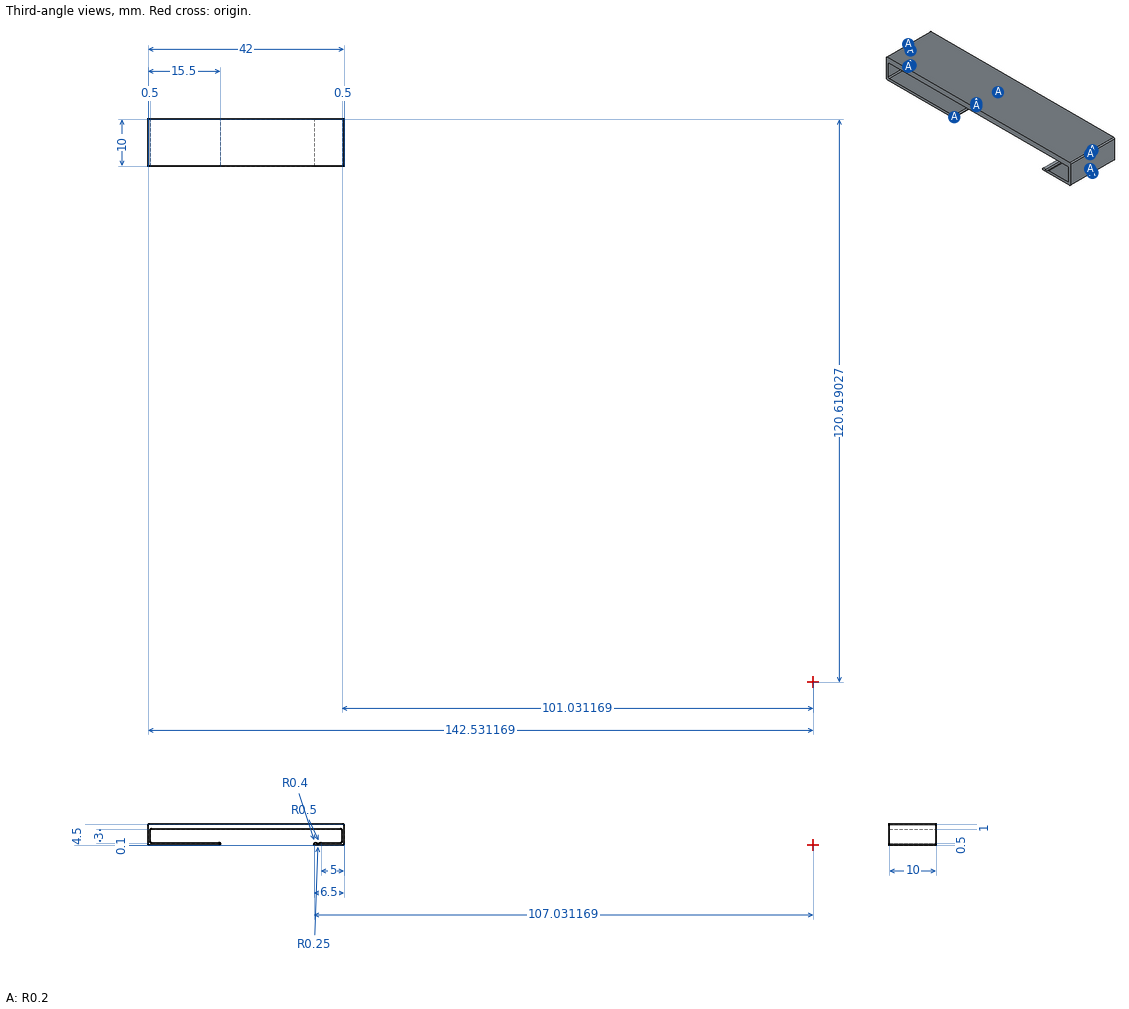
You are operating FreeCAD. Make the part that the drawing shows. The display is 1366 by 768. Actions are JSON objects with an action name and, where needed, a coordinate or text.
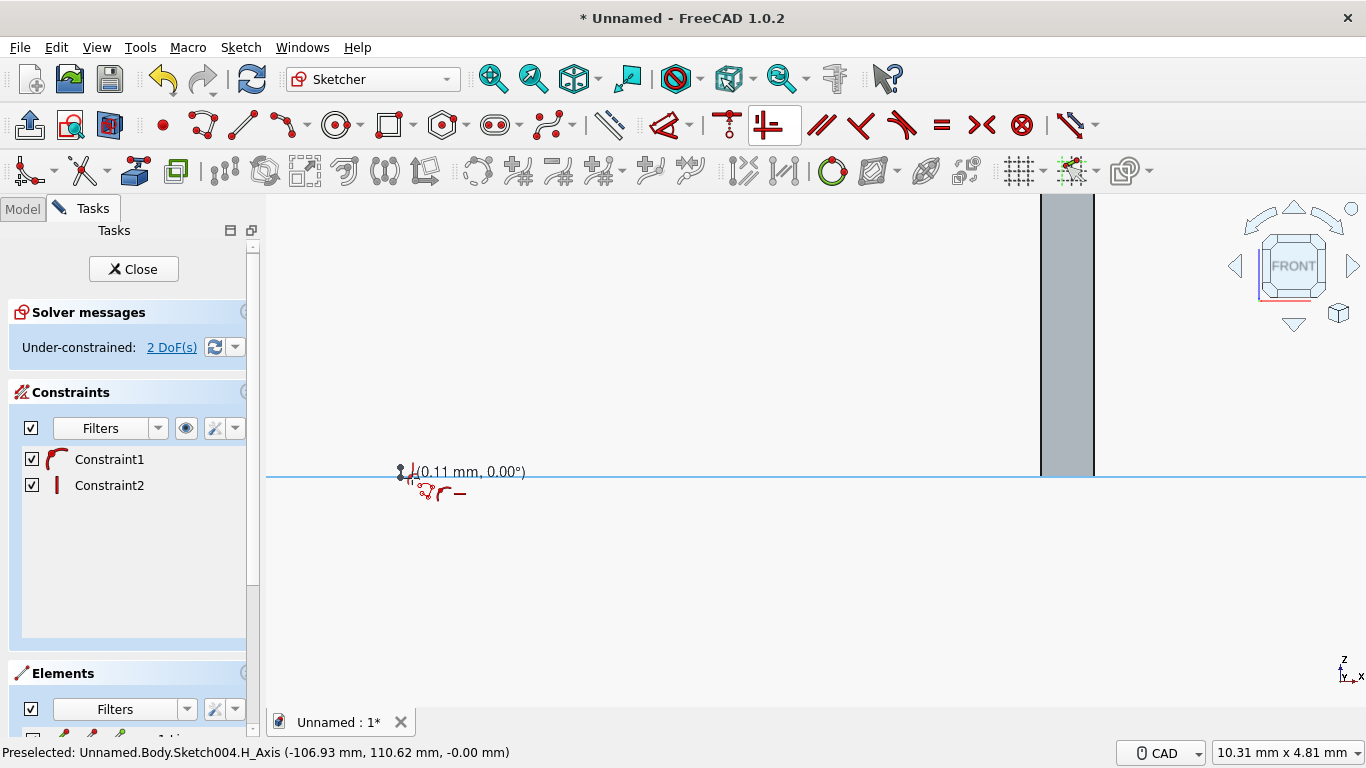
{"action": "left_click", "coordinate": [1094, 468]}
{"action": "left_click", "coordinate": [1094, 424]}
{"action": "left_click", "coordinate": [561, 424]}
{"action": "right_click", "coordinate": [561, 424]}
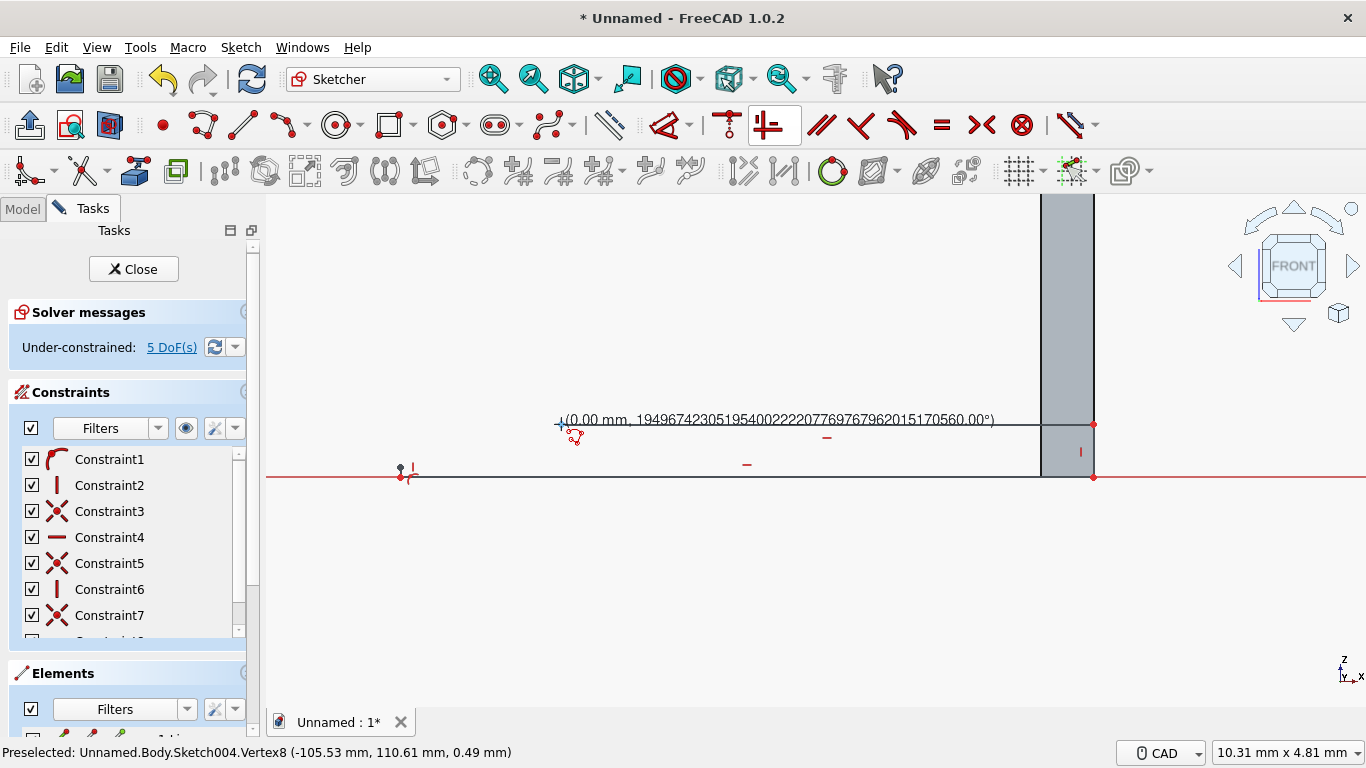
{"action": "left_click", "coordinate": [284, 126]}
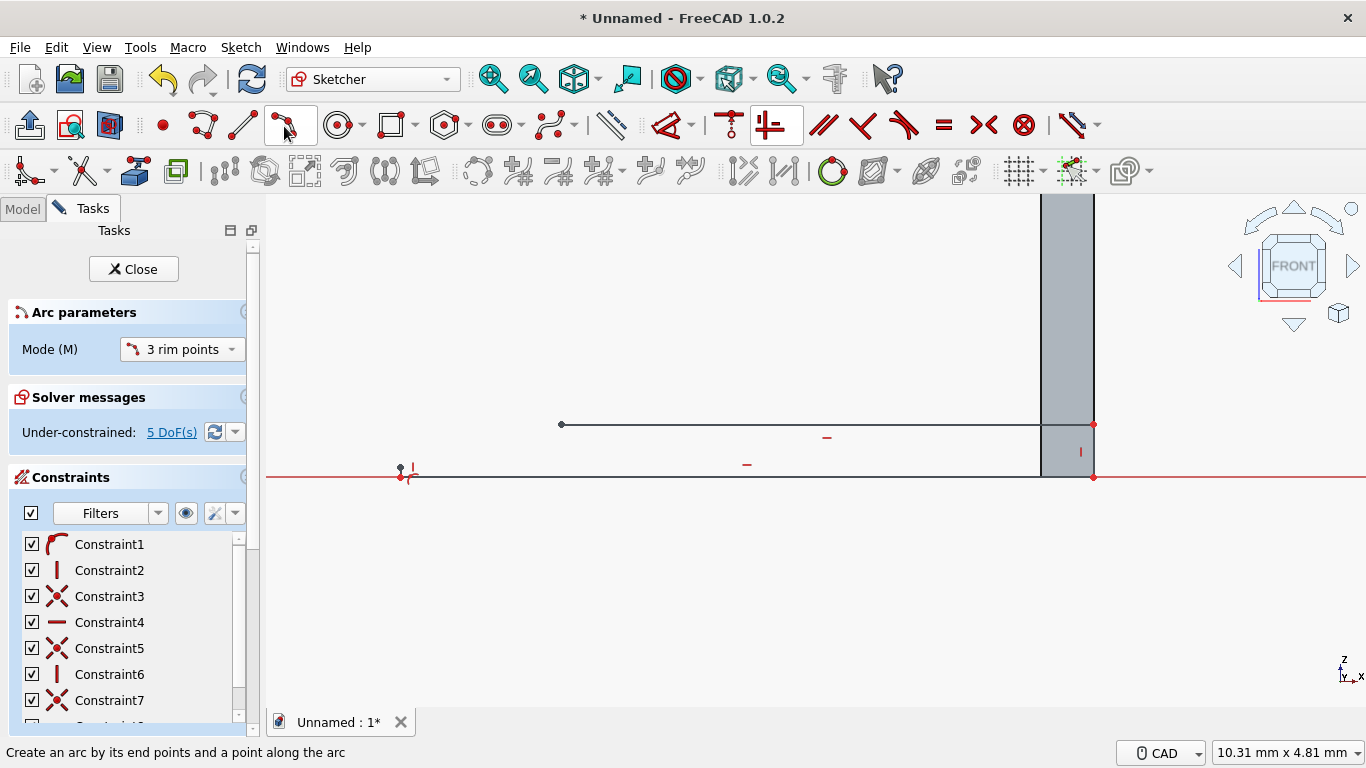
{"action": "left_click", "coordinate": [561, 425]}
{"action": "left_click", "coordinate": [520, 443]}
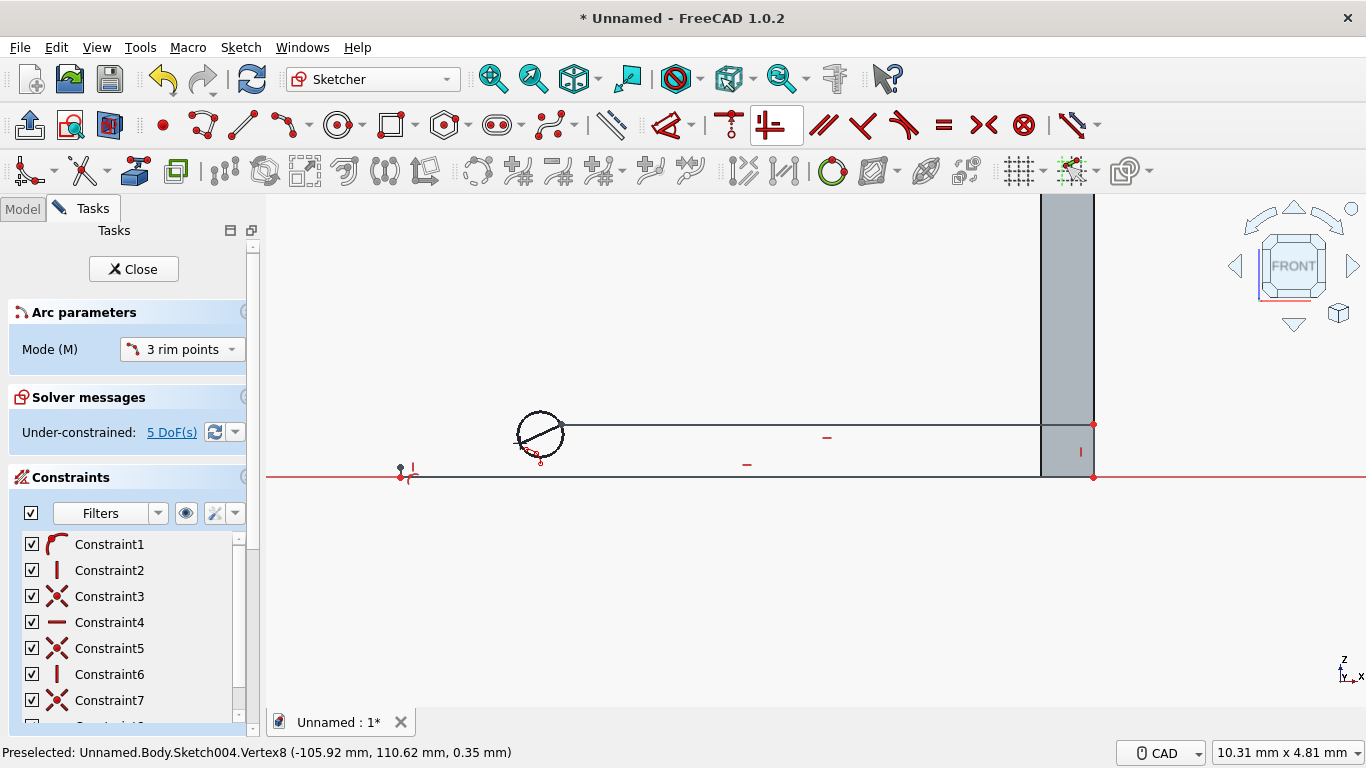
{"action": "scroll", "coordinate": [538, 429], "scroll_direction": "up", "scroll_amount": 6}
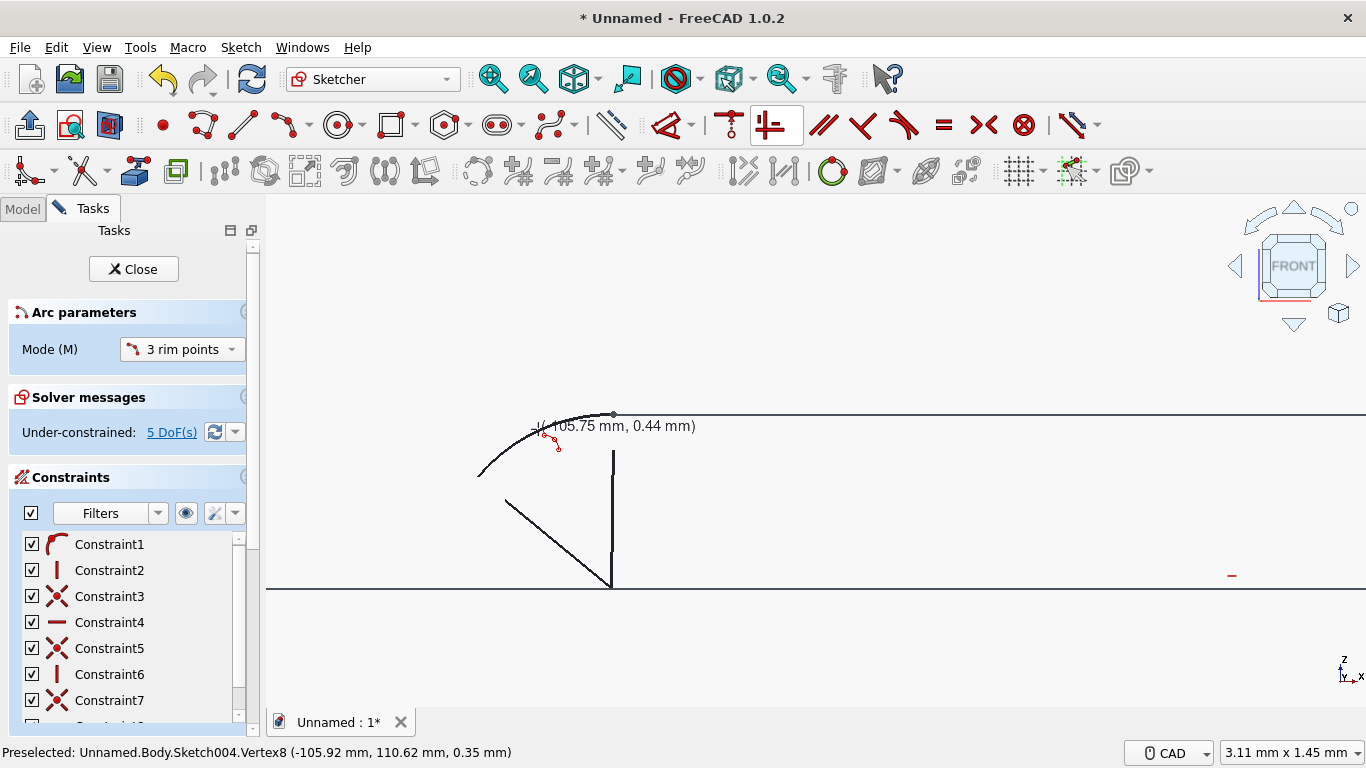
{"action": "left_click", "coordinate": [538, 428]}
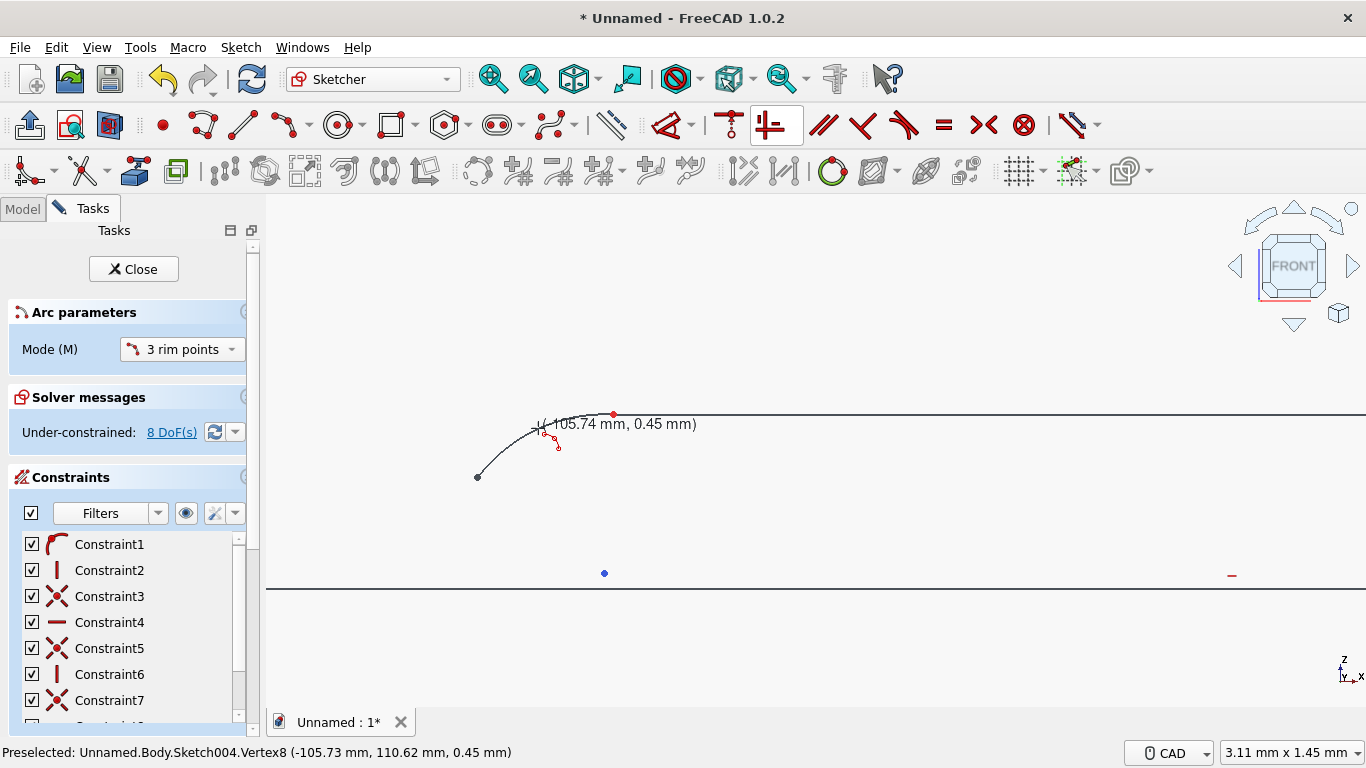
{"action": "left_click", "coordinate": [478, 478]}
{"action": "left_click", "coordinate": [338, 470]}
{"action": "left_click", "coordinate": [407, 506]}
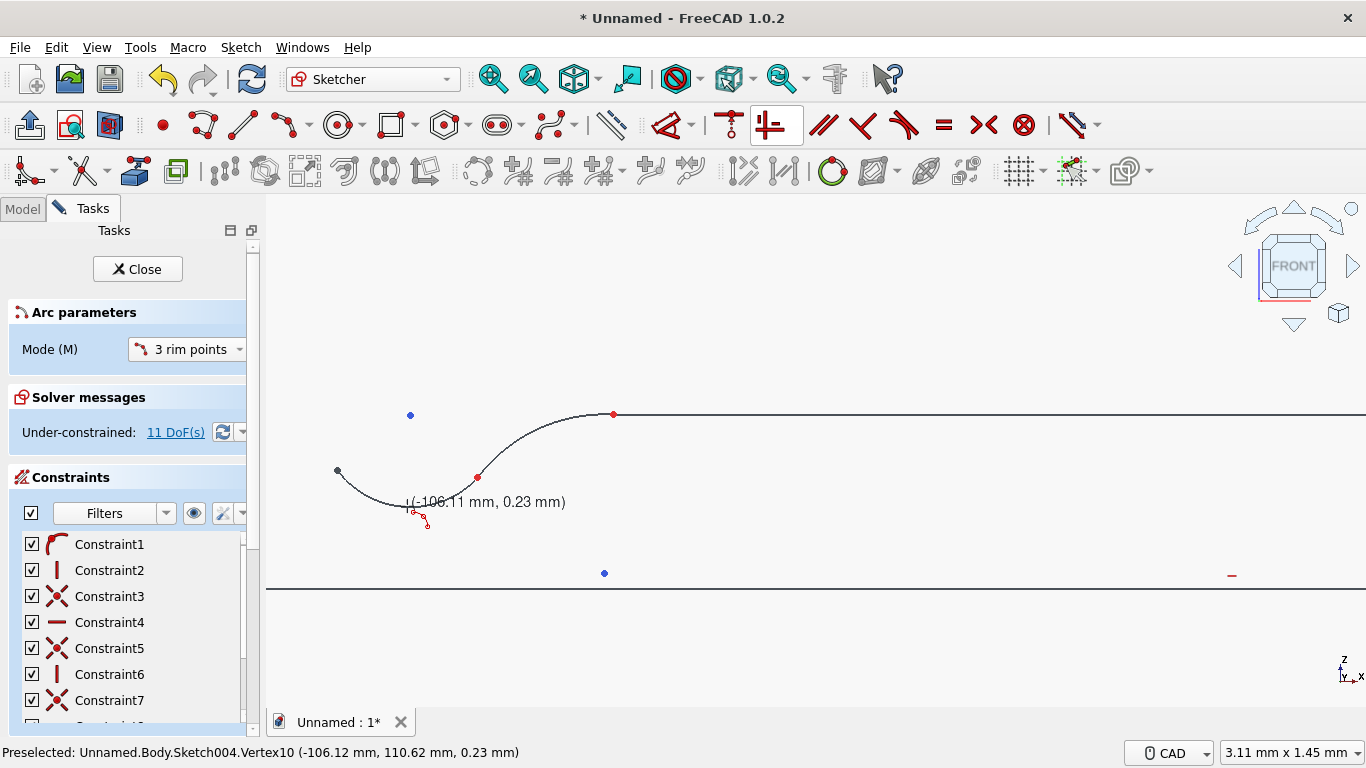
{"action": "left_click", "coordinate": [338, 471]}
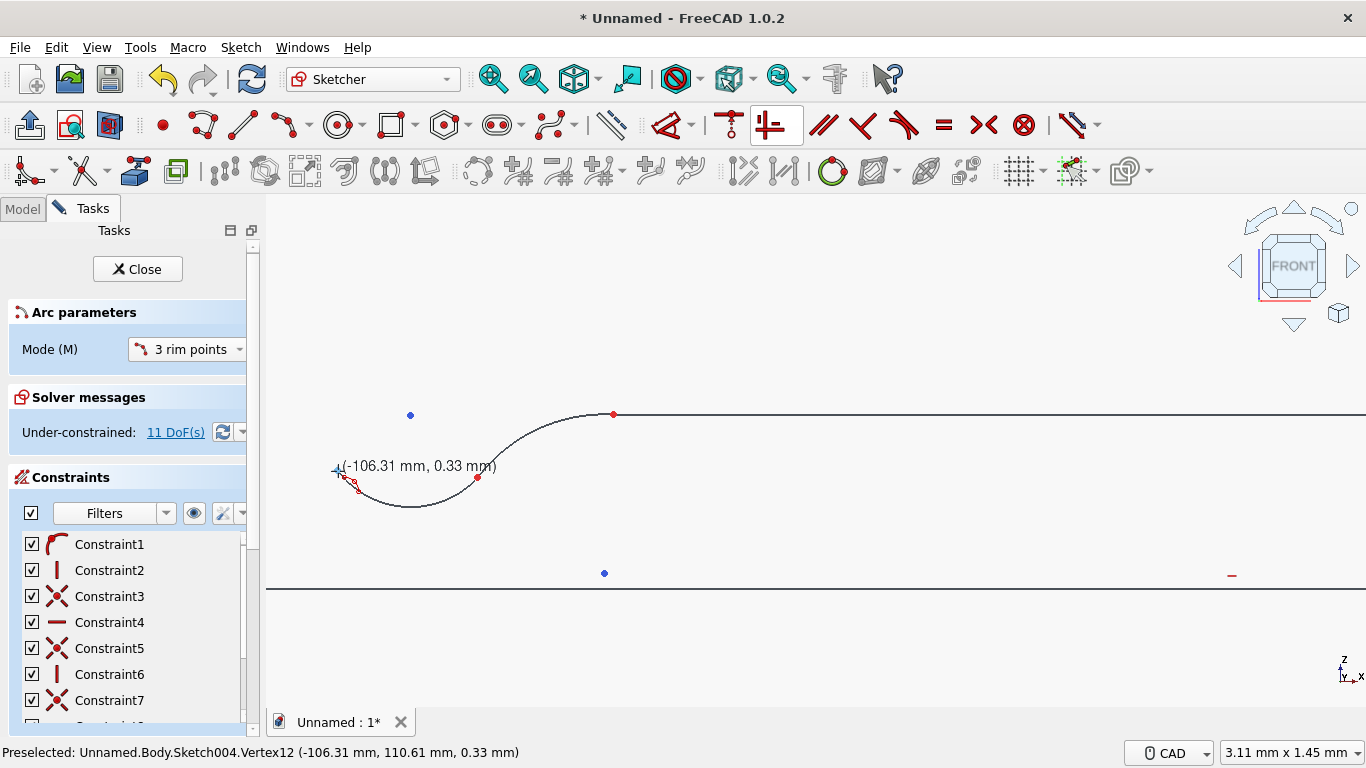
{"action": "scroll", "coordinate": [538, 429], "scroll_direction": "down", "scroll_amount": 6}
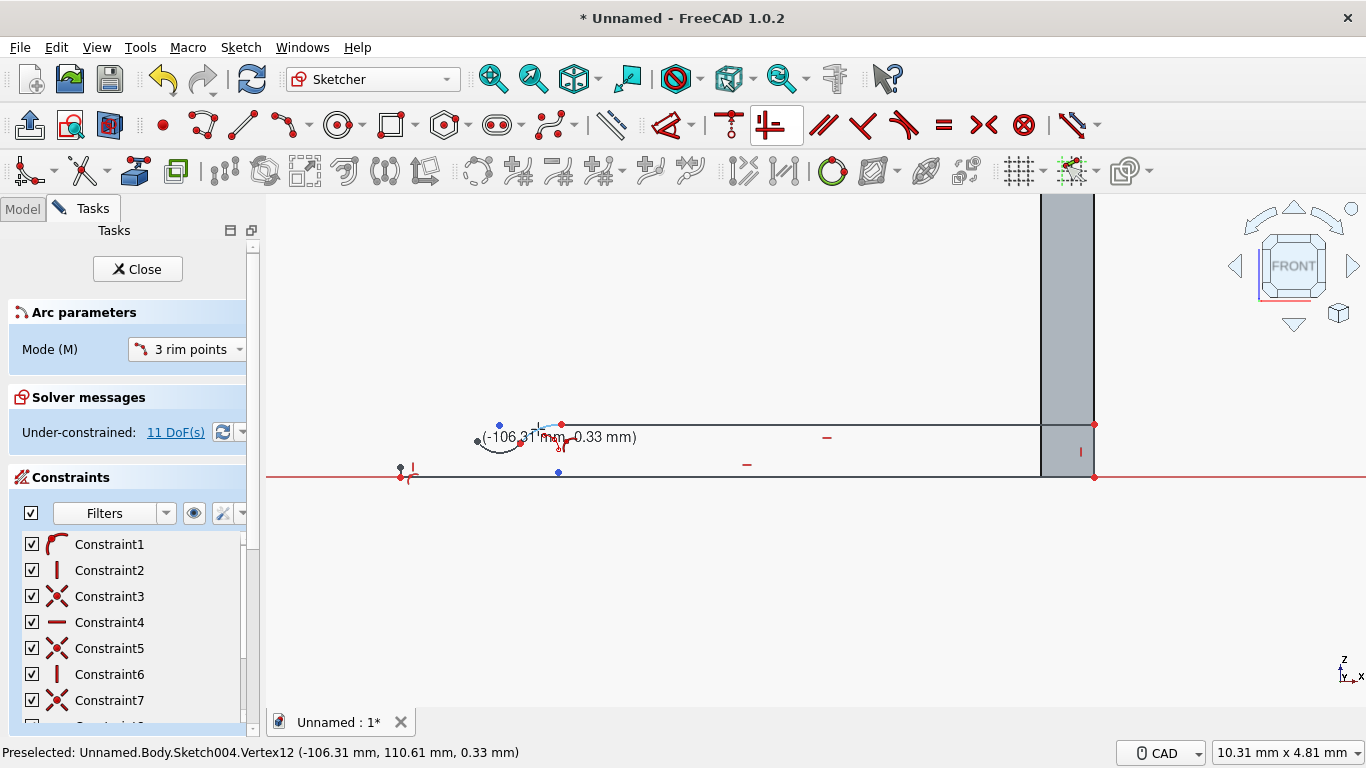
{"action": "scroll", "coordinate": [401, 467], "scroll_direction": "up", "scroll_amount": 6}